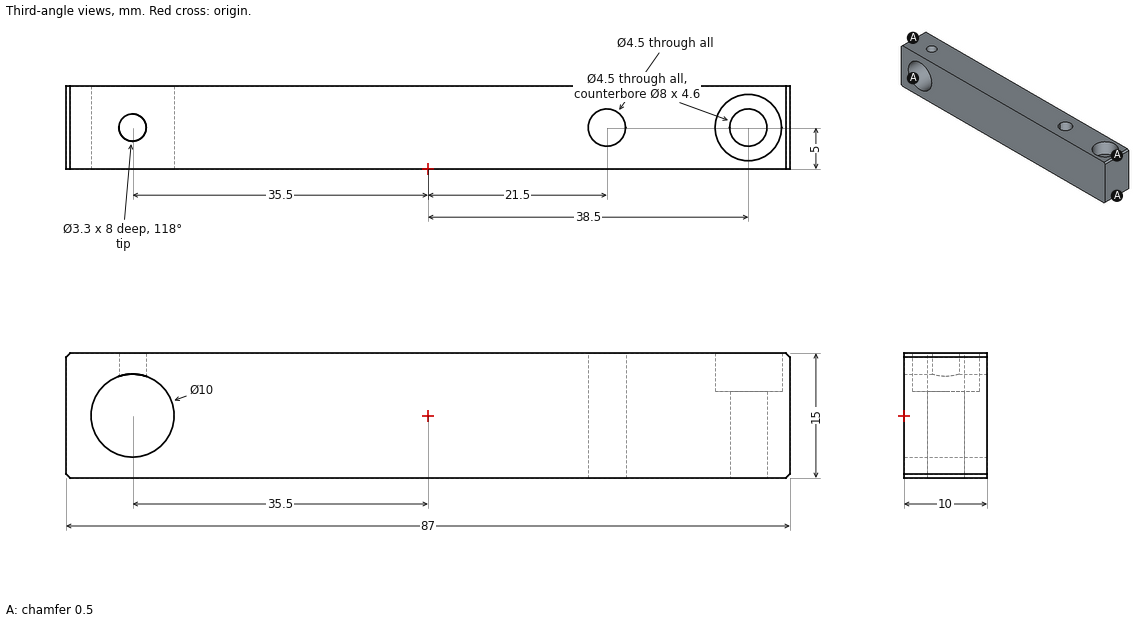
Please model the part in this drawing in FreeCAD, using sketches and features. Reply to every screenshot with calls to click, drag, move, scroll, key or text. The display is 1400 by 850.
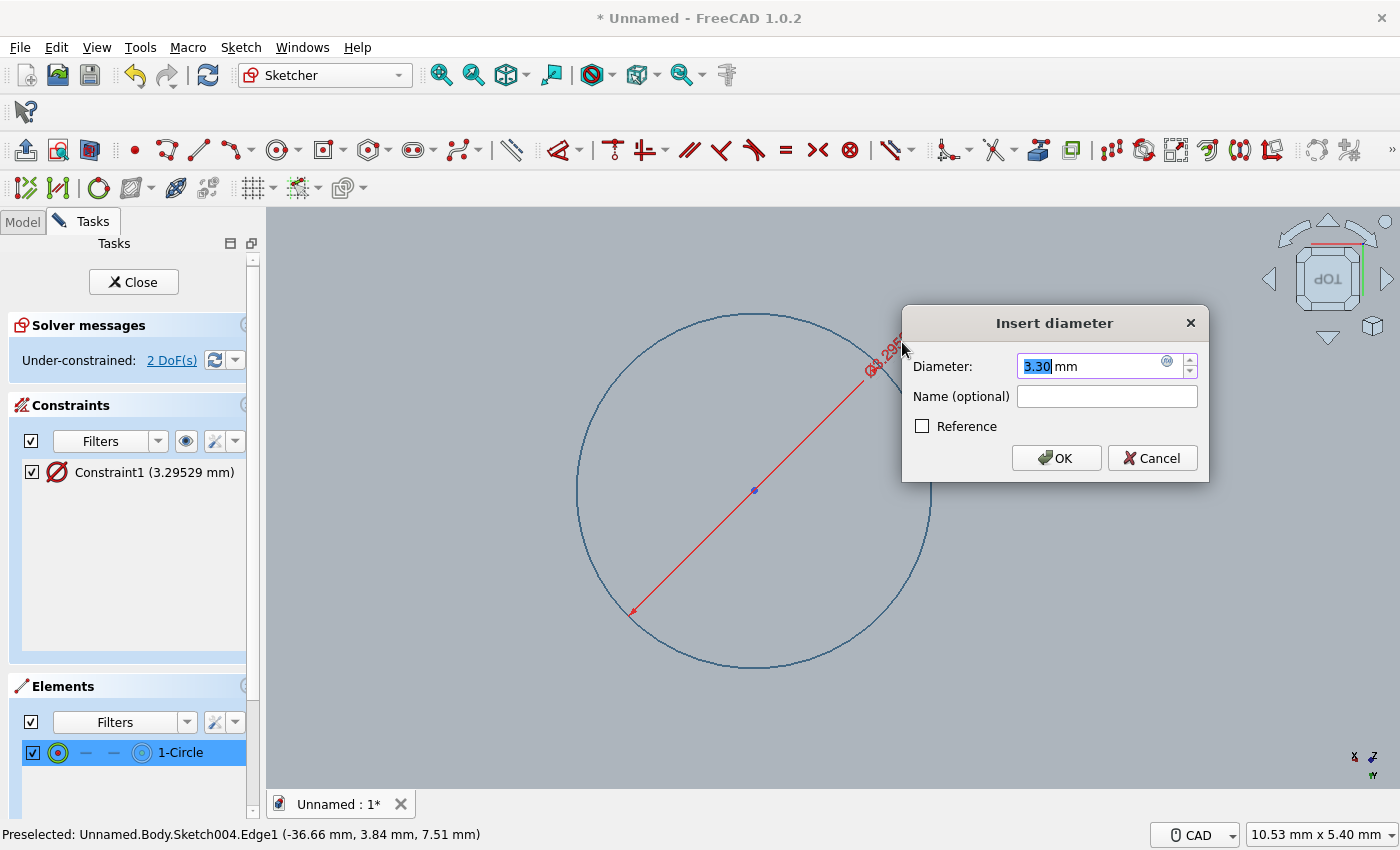
text(3.3)
key(Return)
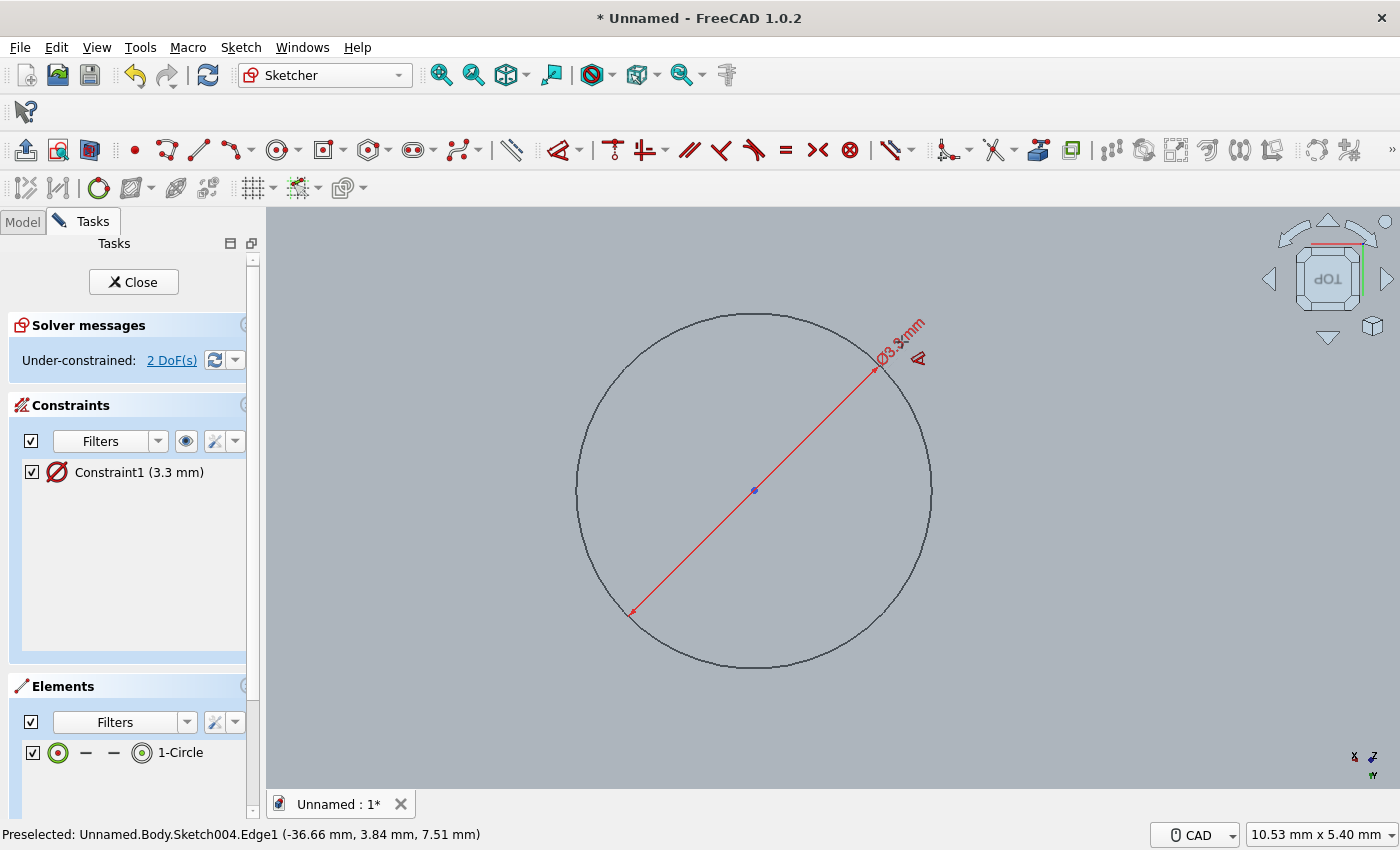
click(754, 491)
click(788, 363)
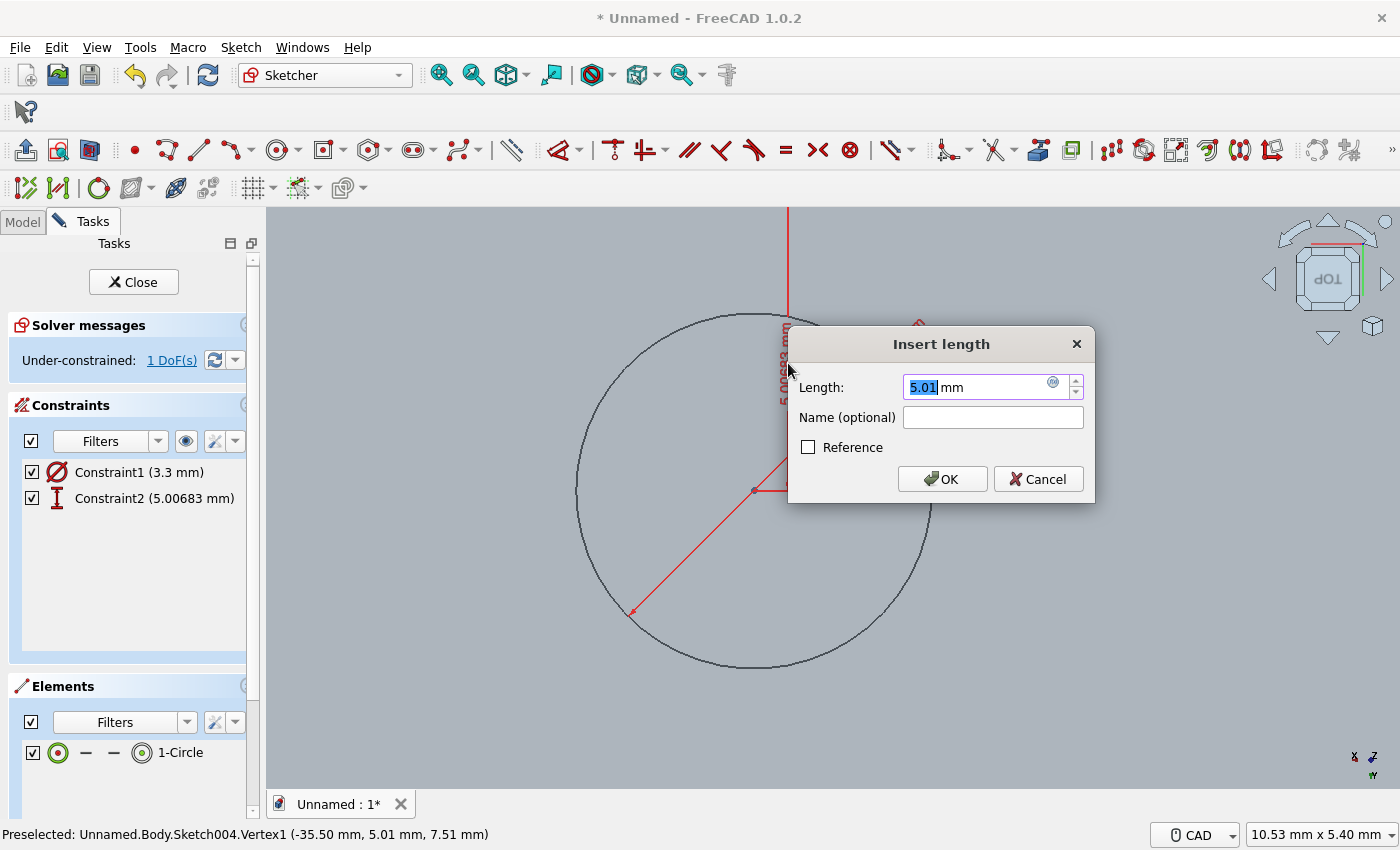
text(5)
key(Return)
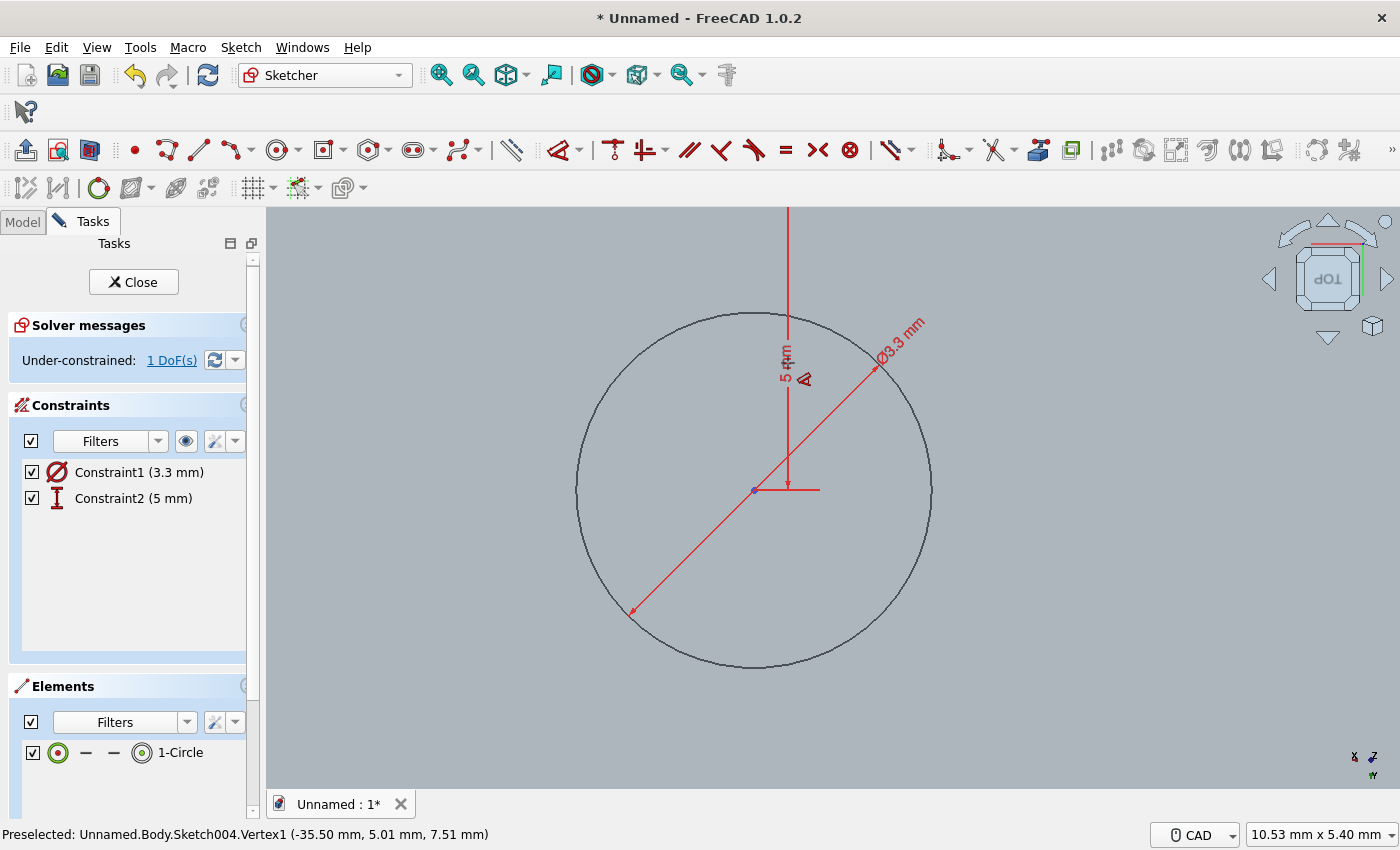
click(754, 490)
click(524, 524)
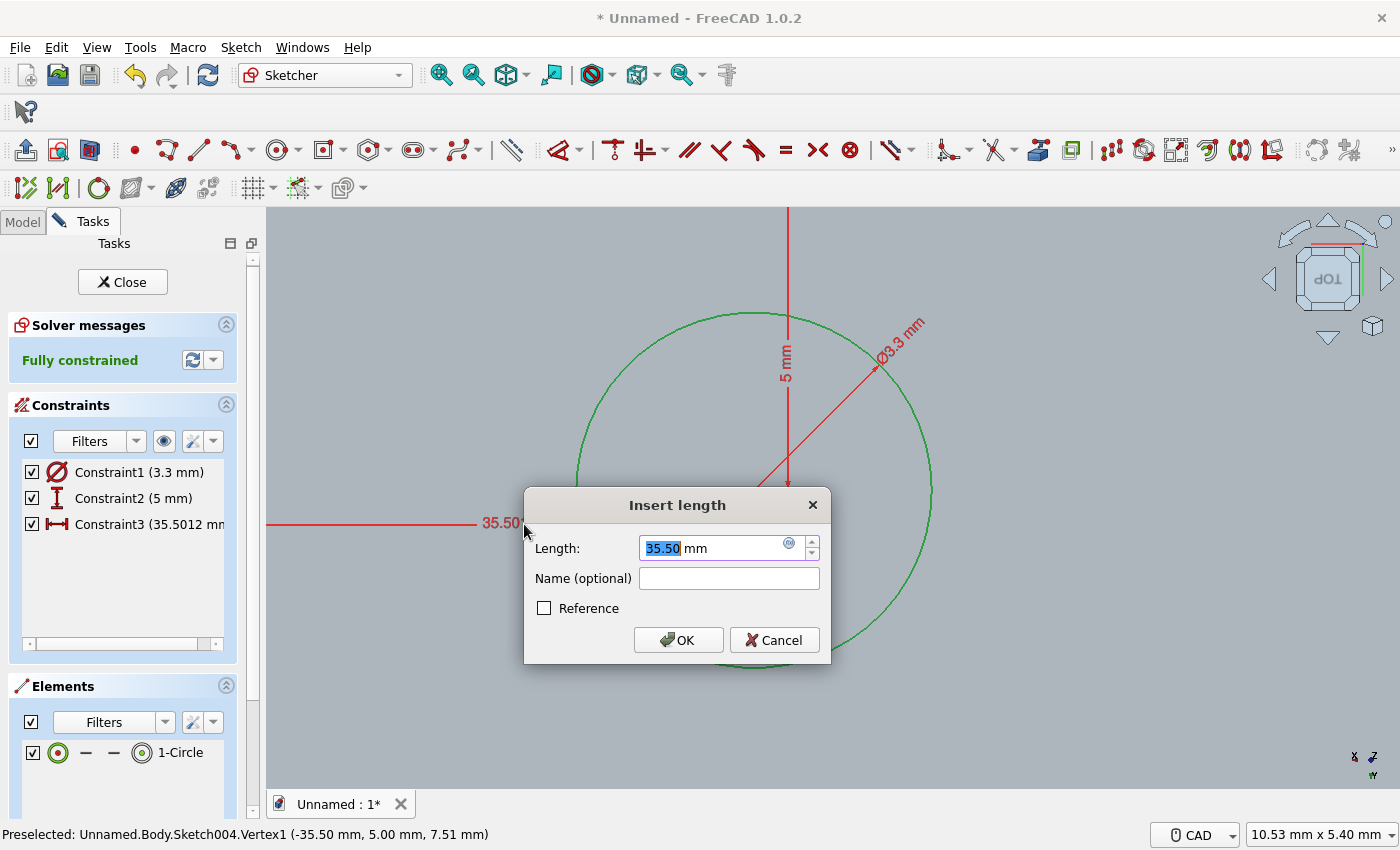
text(35.5)
key(Return)
key(Escape)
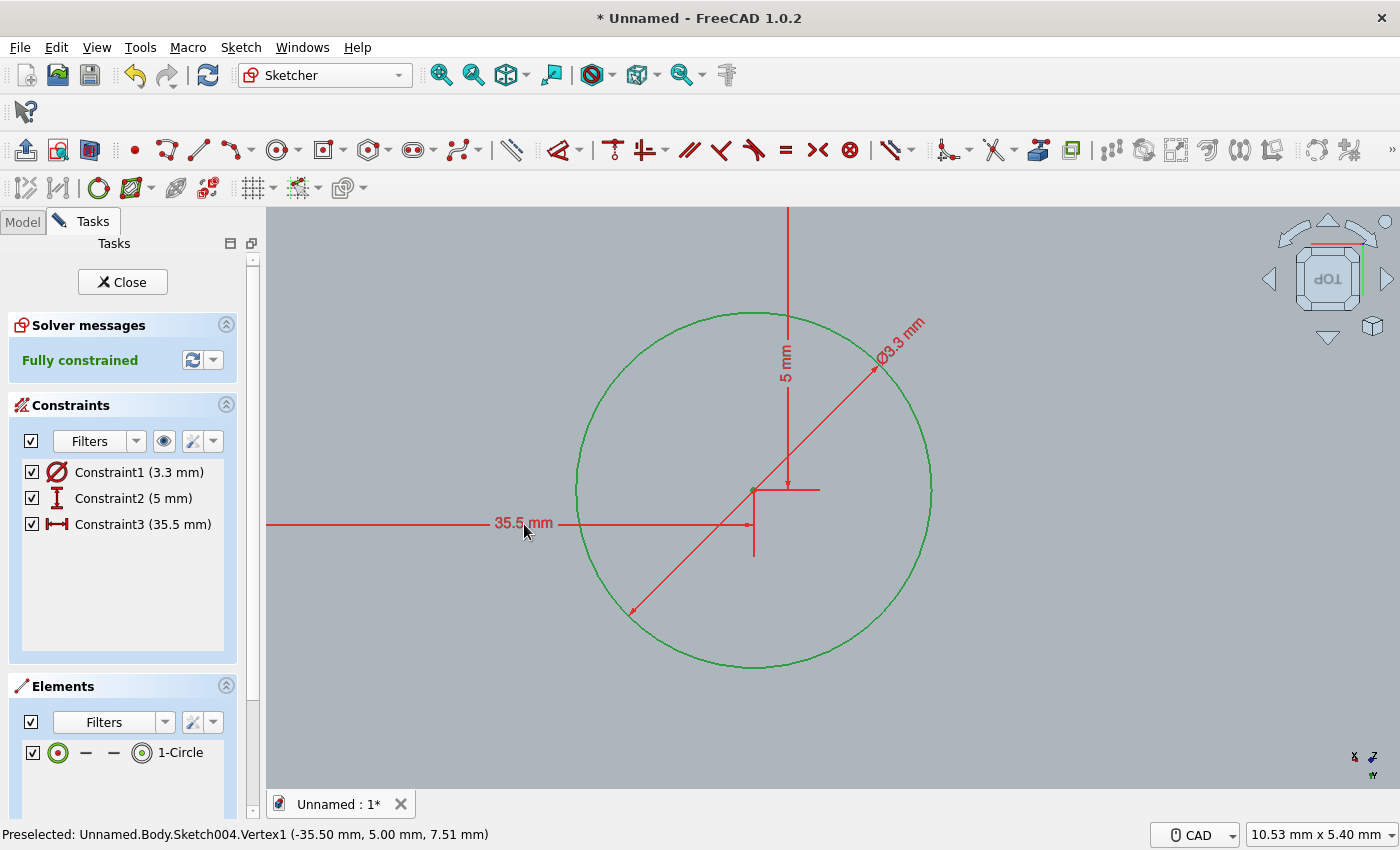
click(123, 282)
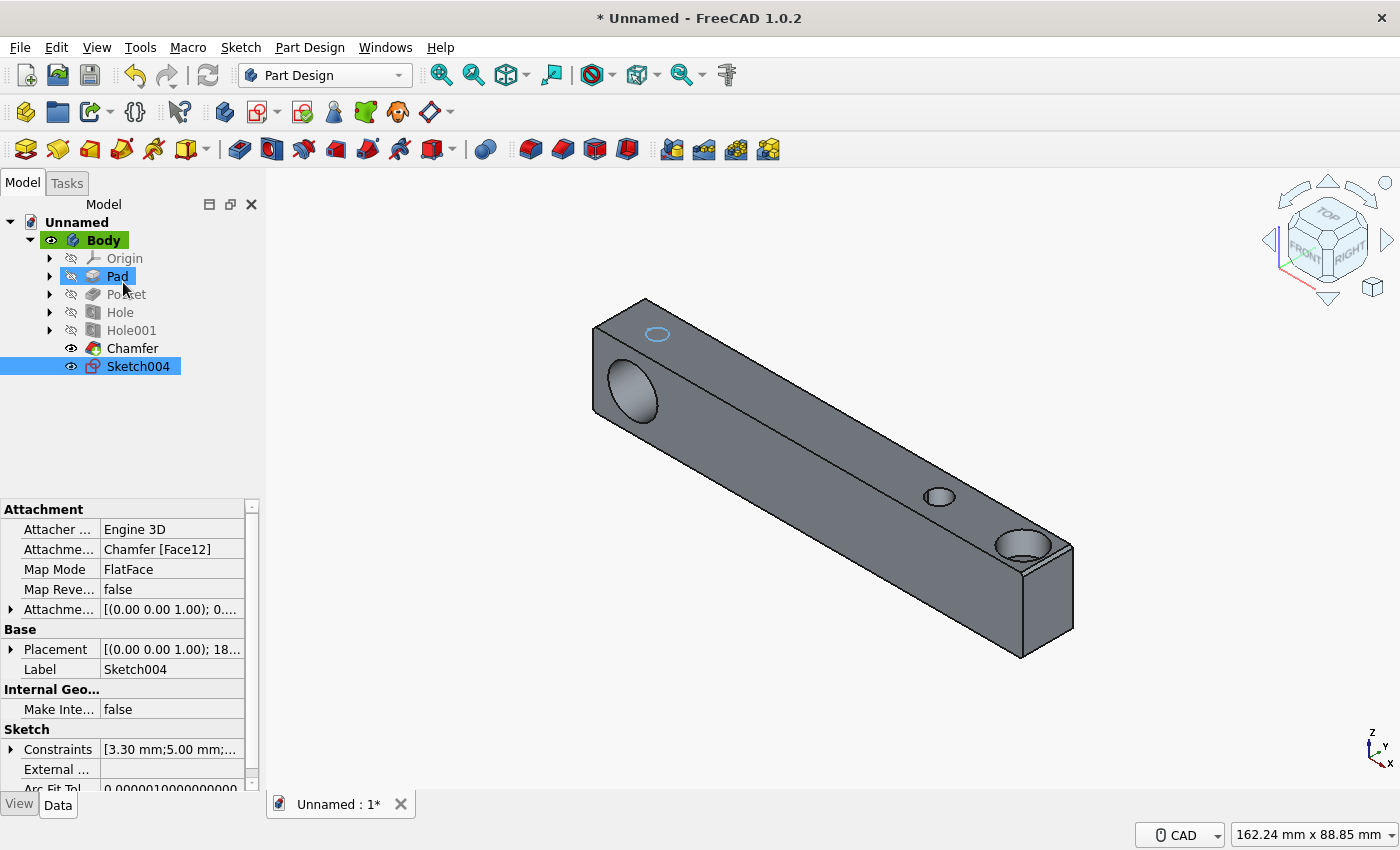
click(272, 150)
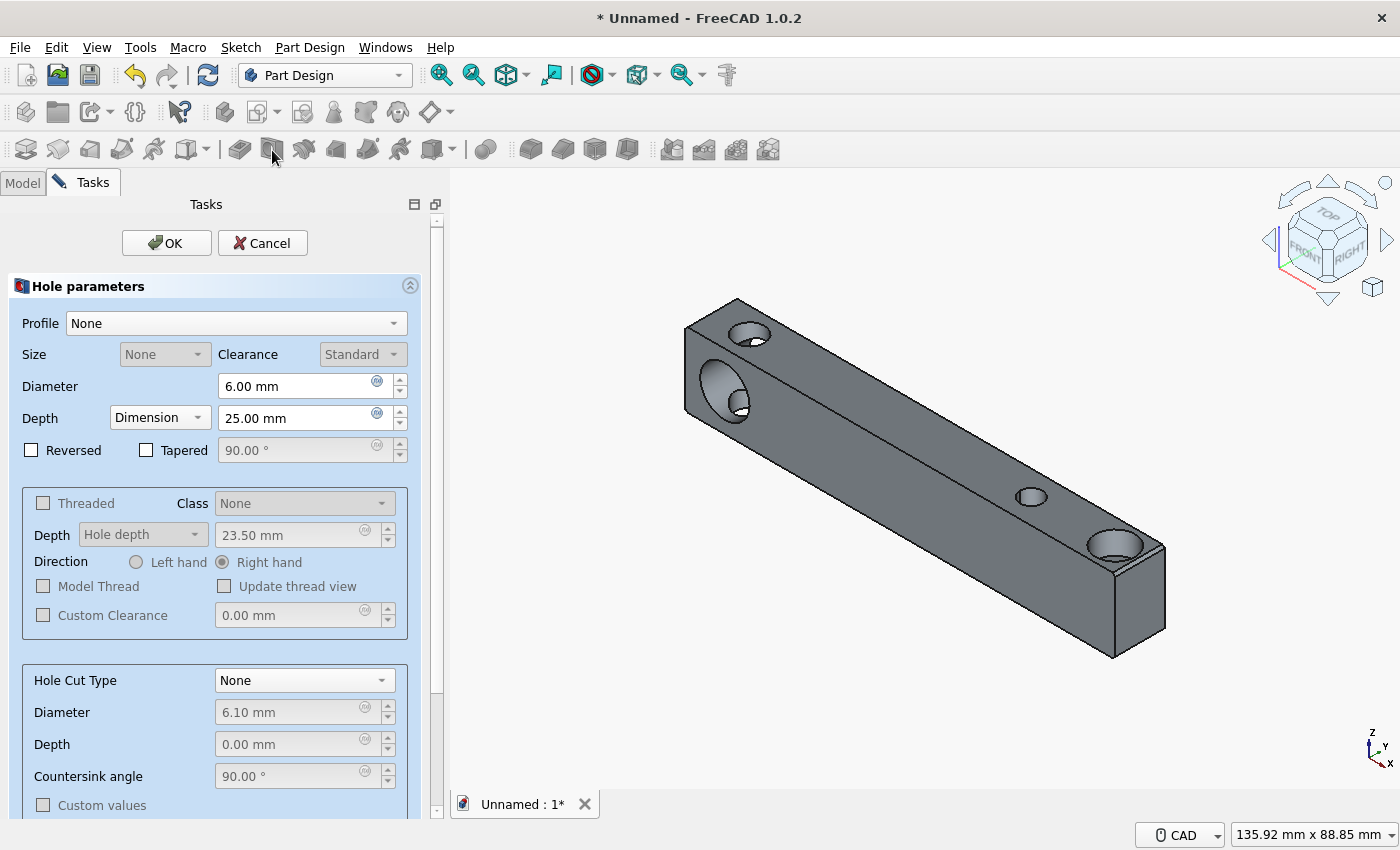
triple_click(305, 386)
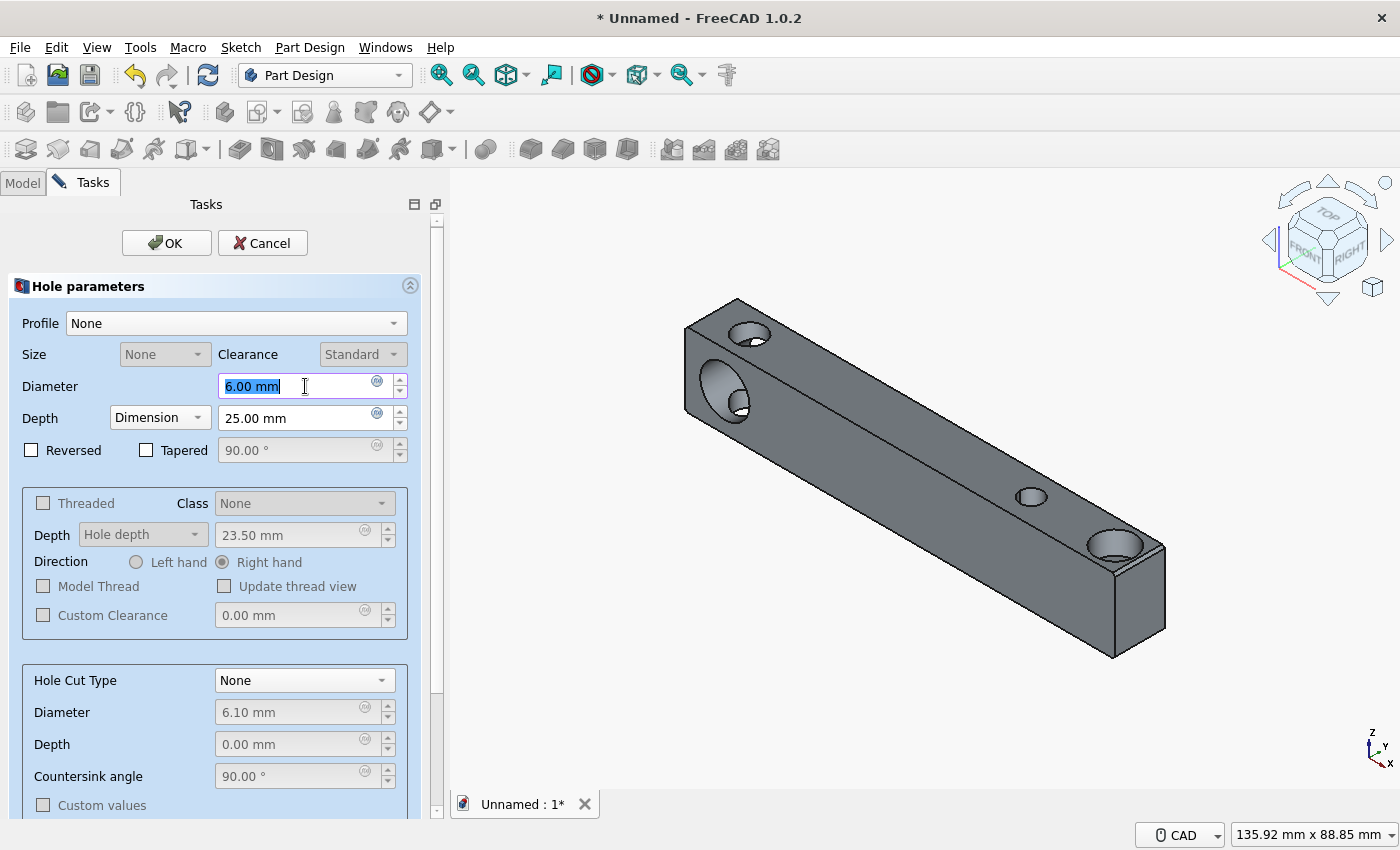
text(3.3)
key(Tab)